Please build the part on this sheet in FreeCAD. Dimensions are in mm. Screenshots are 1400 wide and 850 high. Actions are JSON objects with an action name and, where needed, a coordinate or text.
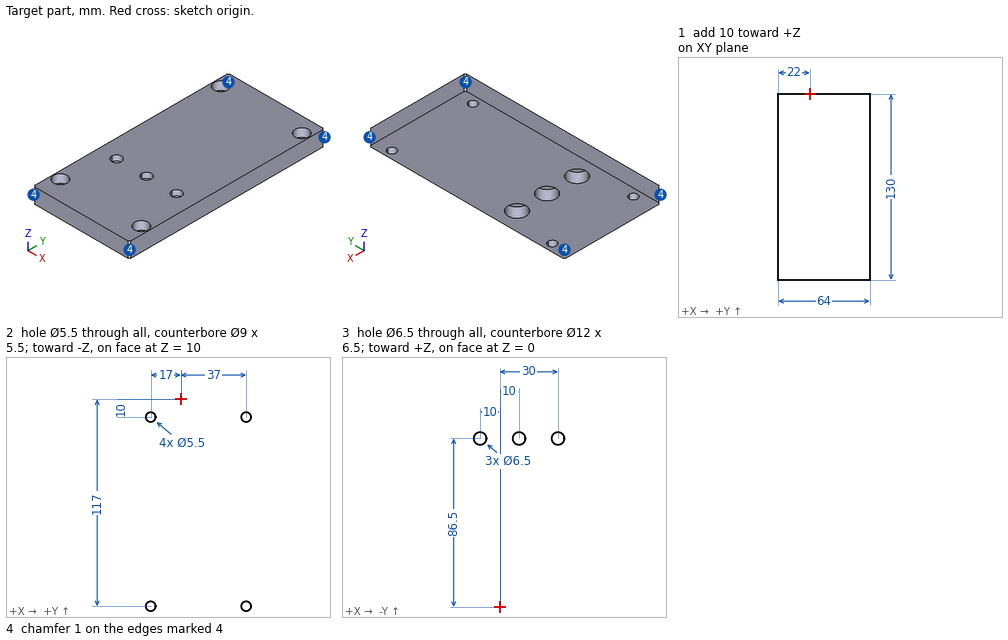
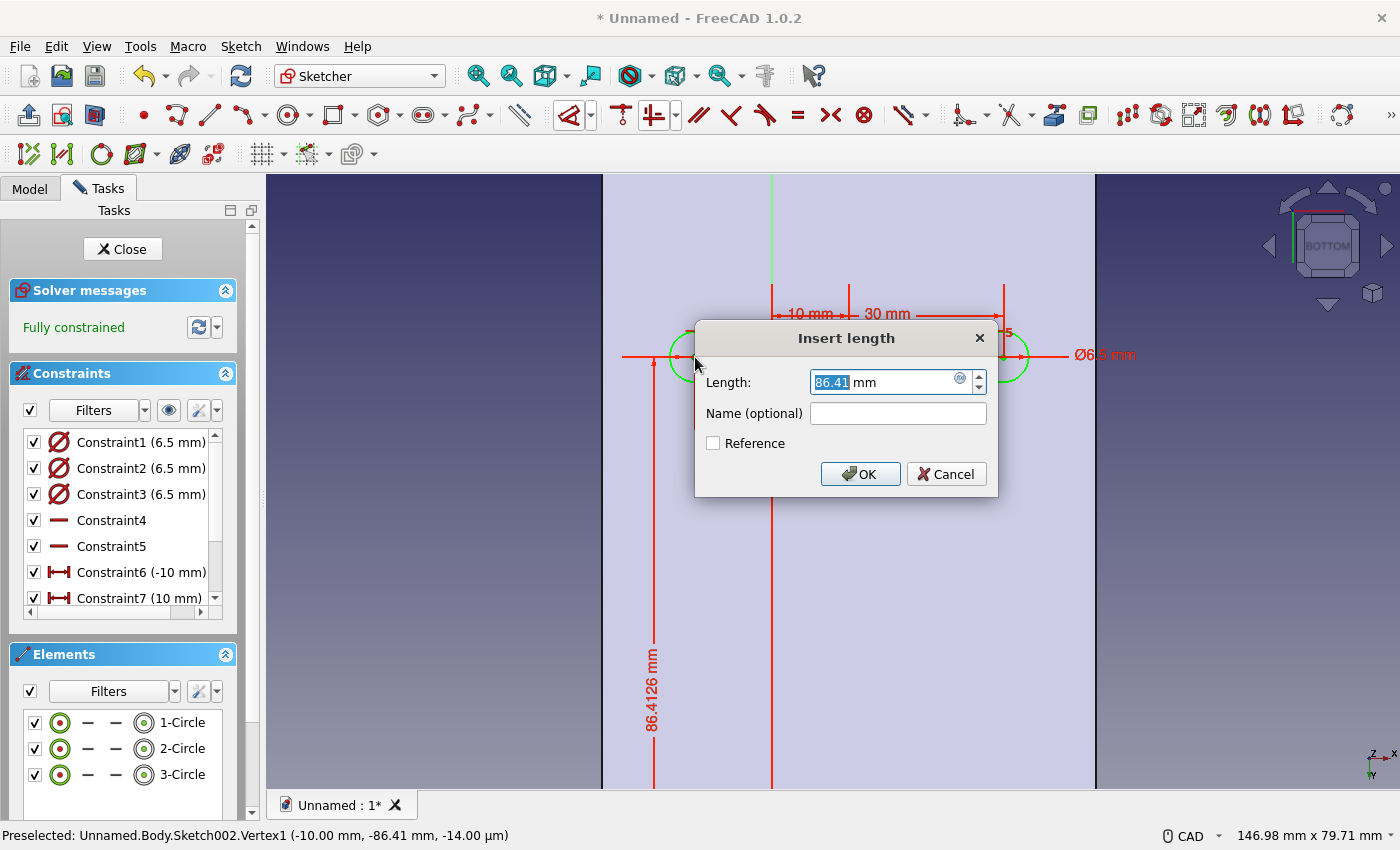
{"action": "type", "text": "86.5"}
{"action": "key", "text": "Return"}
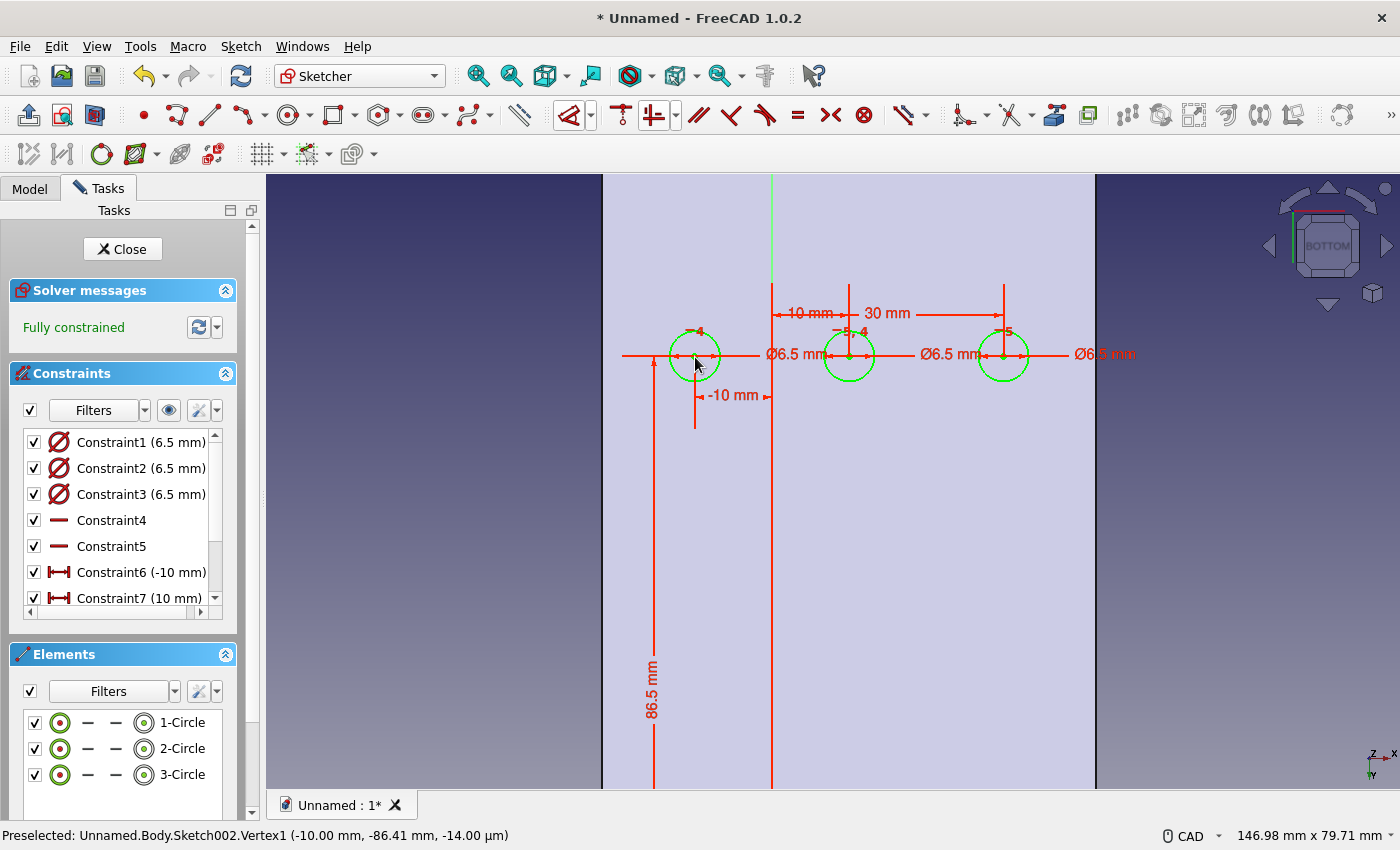
{"action": "left_click", "coordinate": [123, 249]}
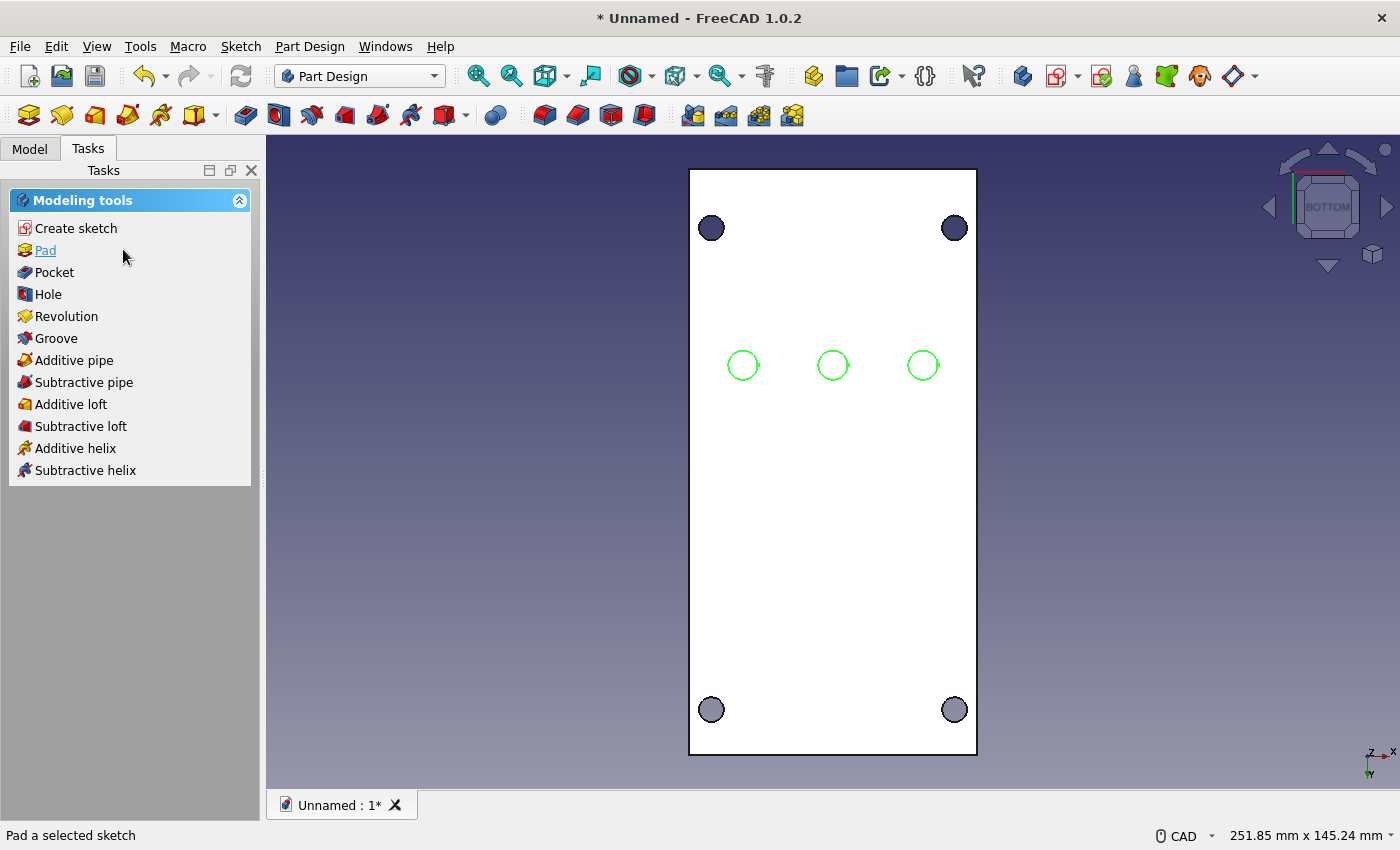
{"action": "left_click", "coordinate": [279, 116]}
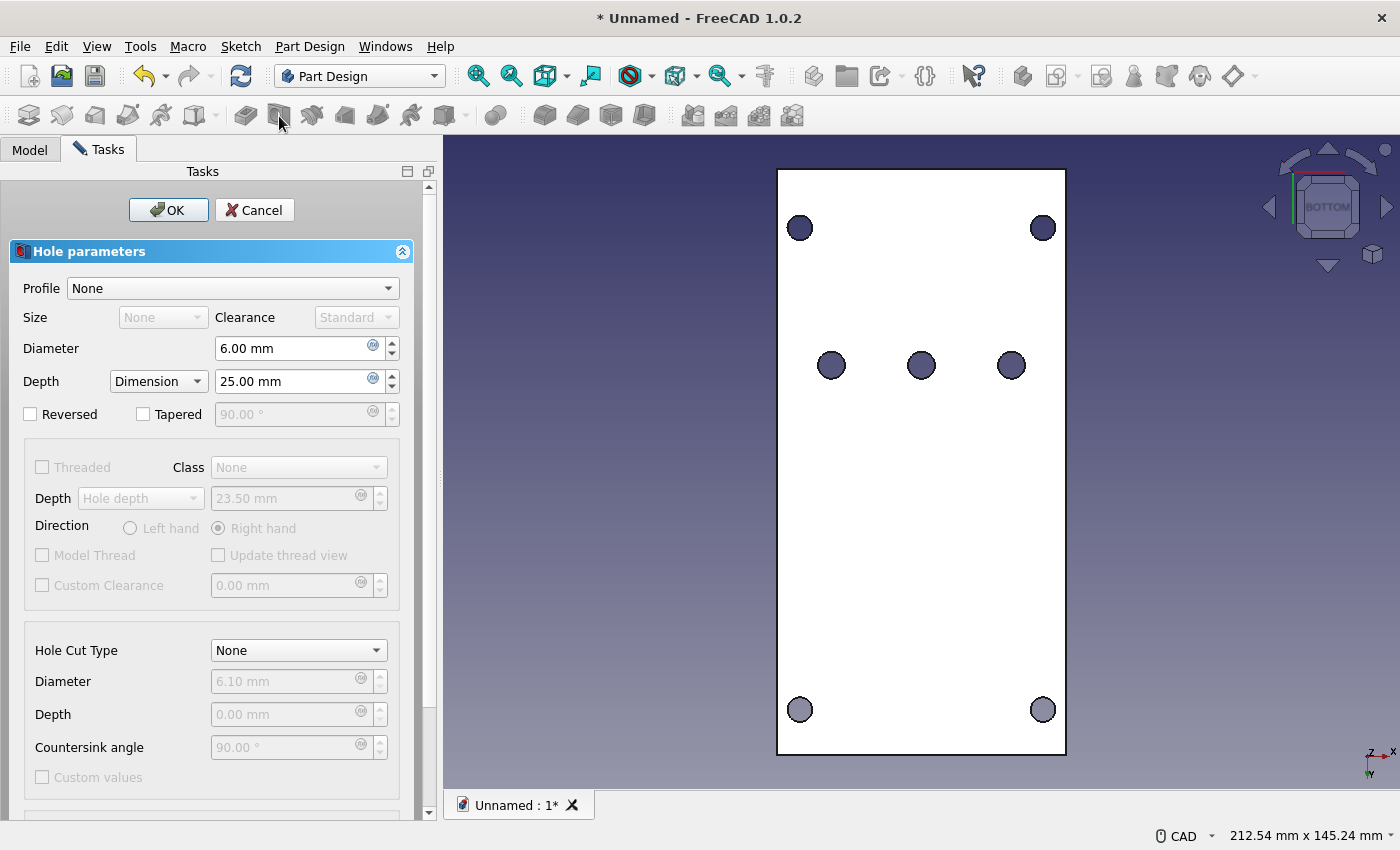
{"action": "triple_click", "coordinate": [300, 348]}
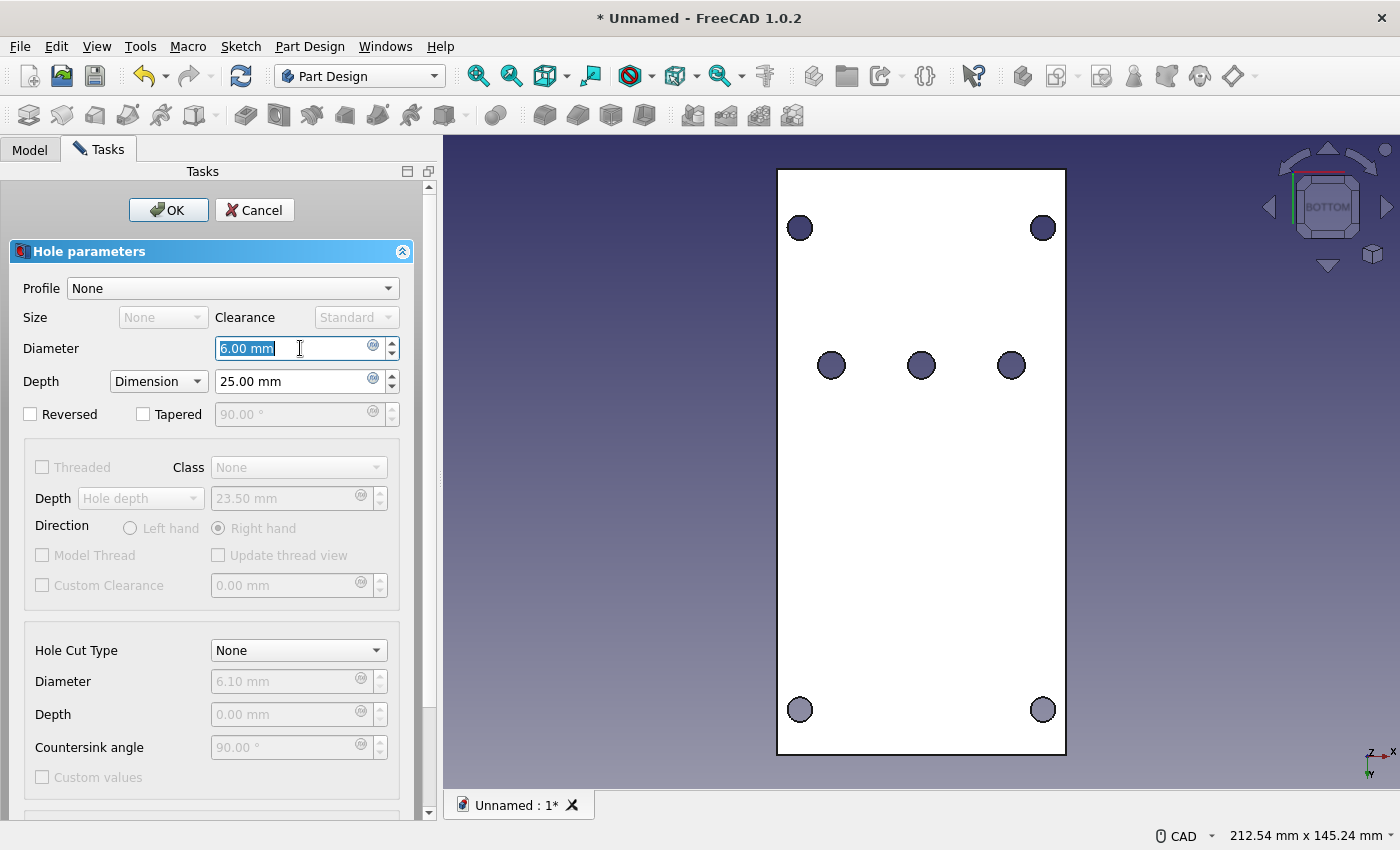
{"action": "type", "text": "6.5"}
{"action": "key", "text": "Tab"}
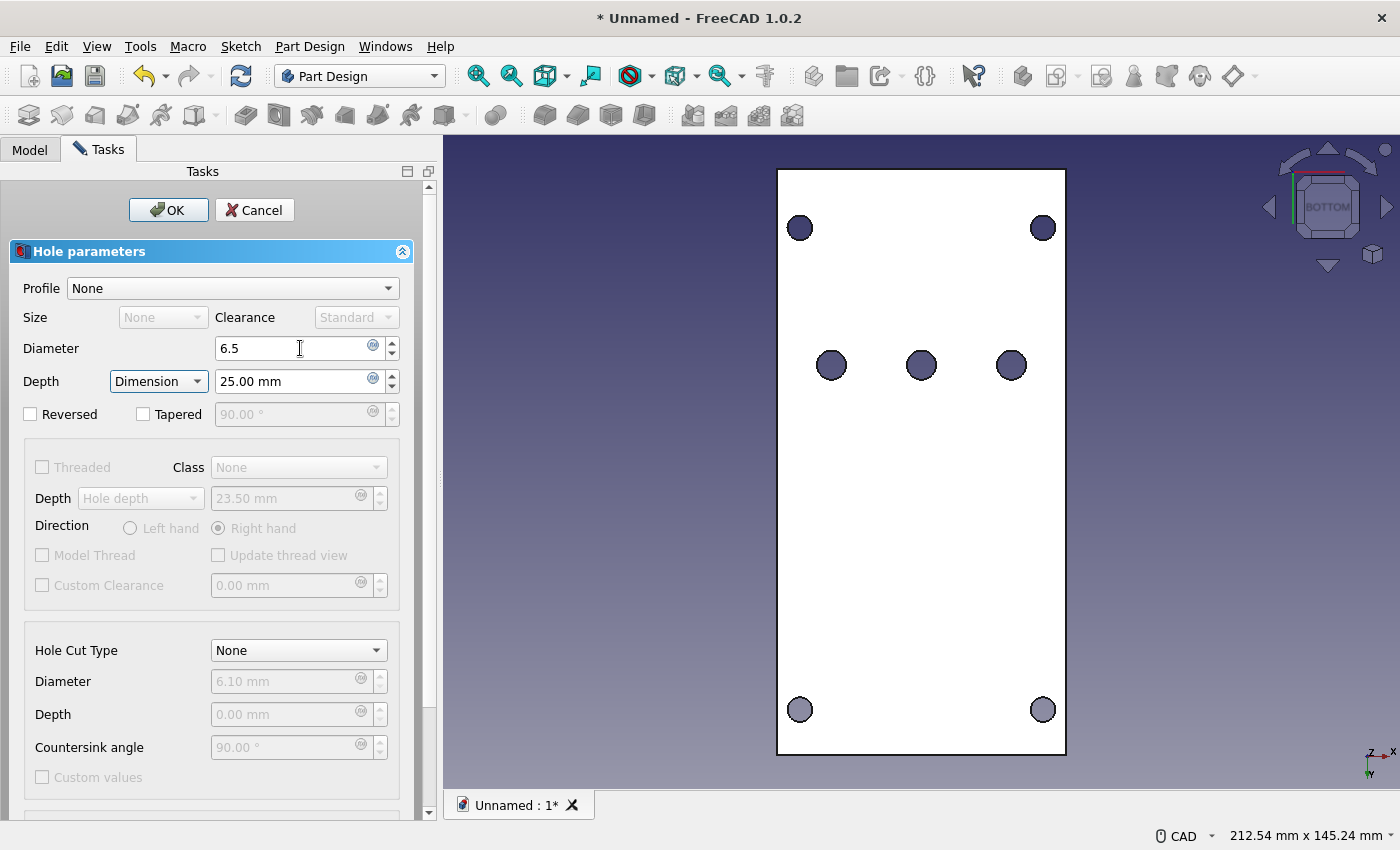
{"action": "left_click", "coordinate": [160, 382]}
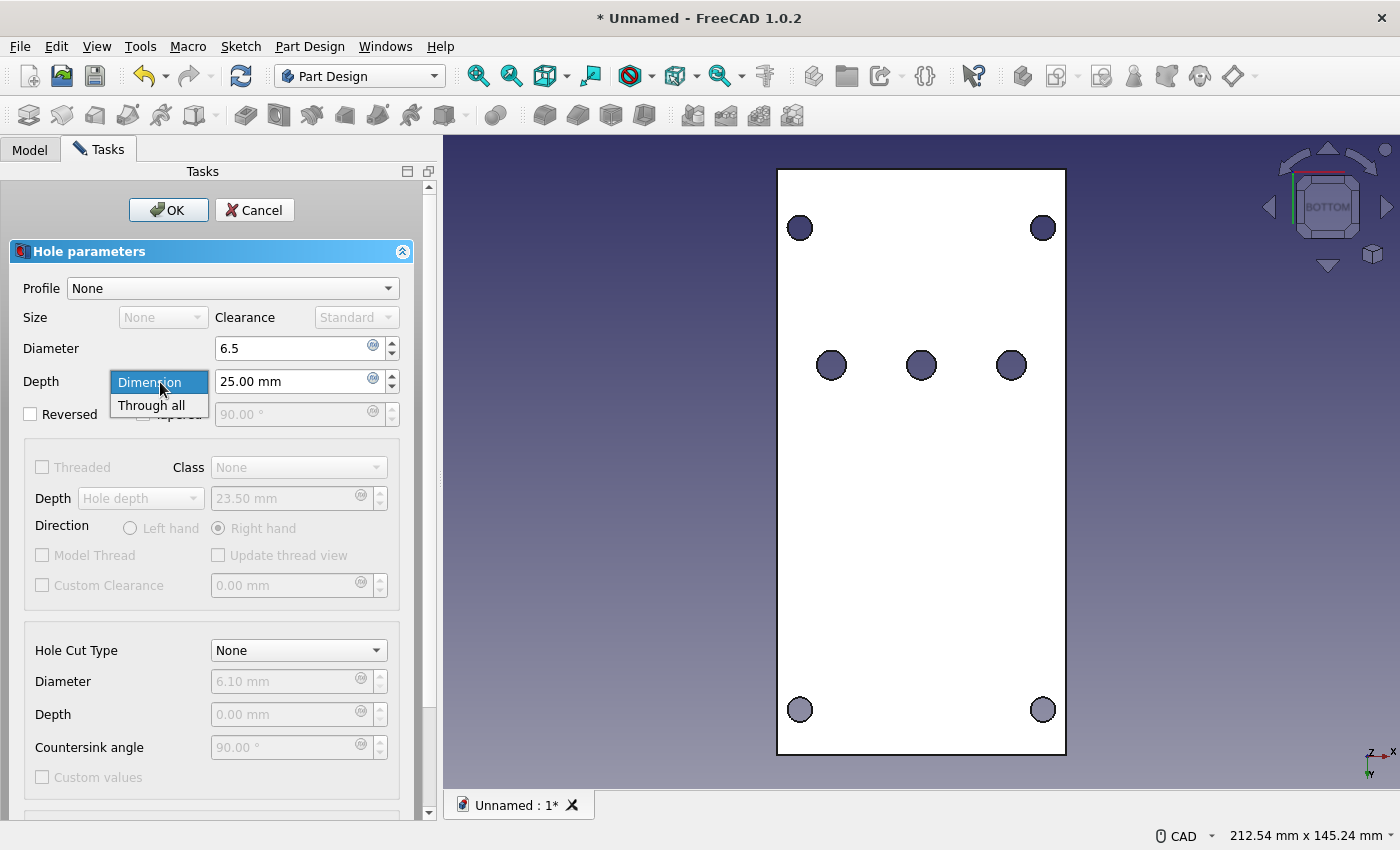
{"action": "left_click", "coordinate": [158, 406]}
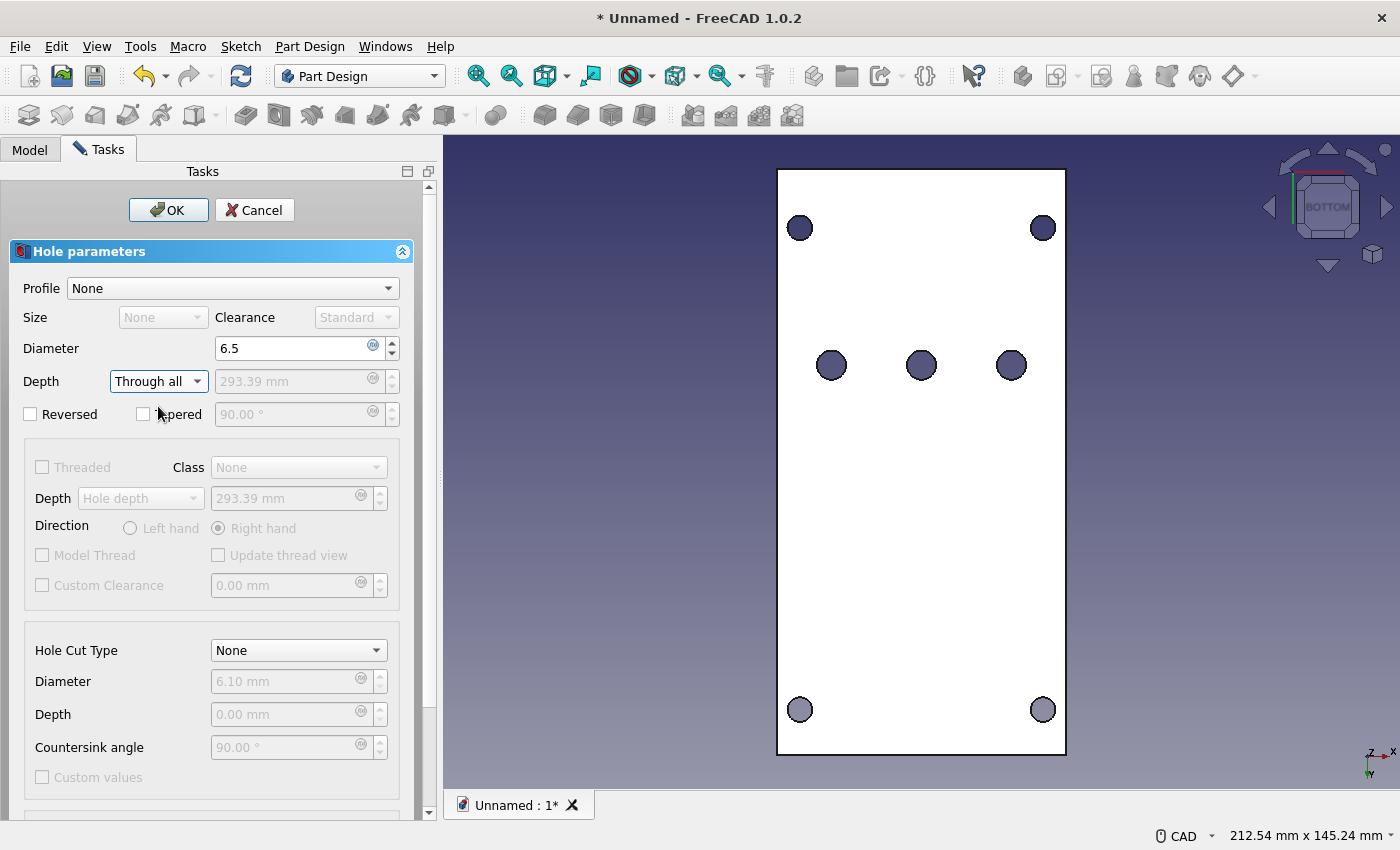
{"action": "left_click", "coordinate": [300, 650]}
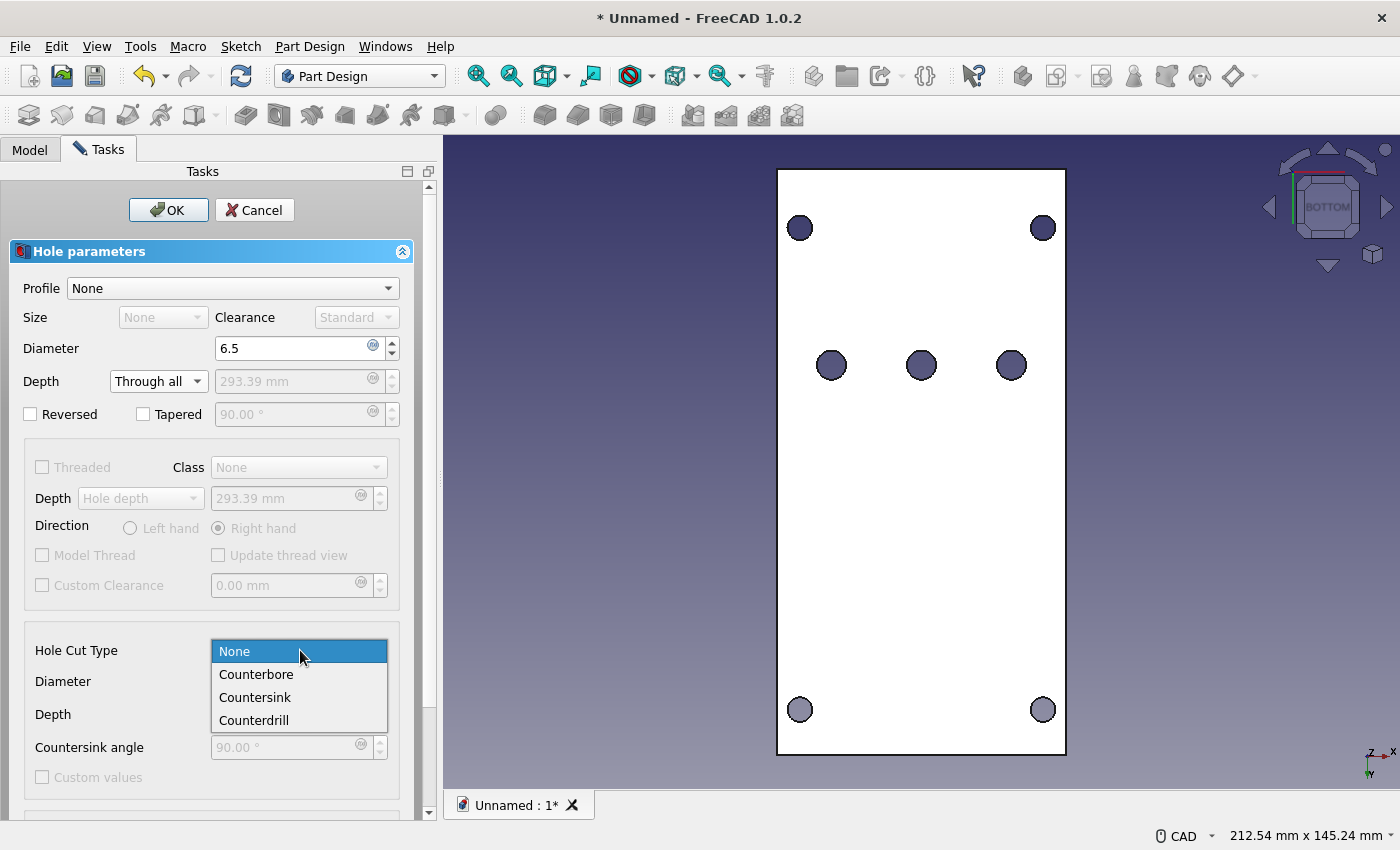
{"action": "left_click", "coordinate": [298, 674]}